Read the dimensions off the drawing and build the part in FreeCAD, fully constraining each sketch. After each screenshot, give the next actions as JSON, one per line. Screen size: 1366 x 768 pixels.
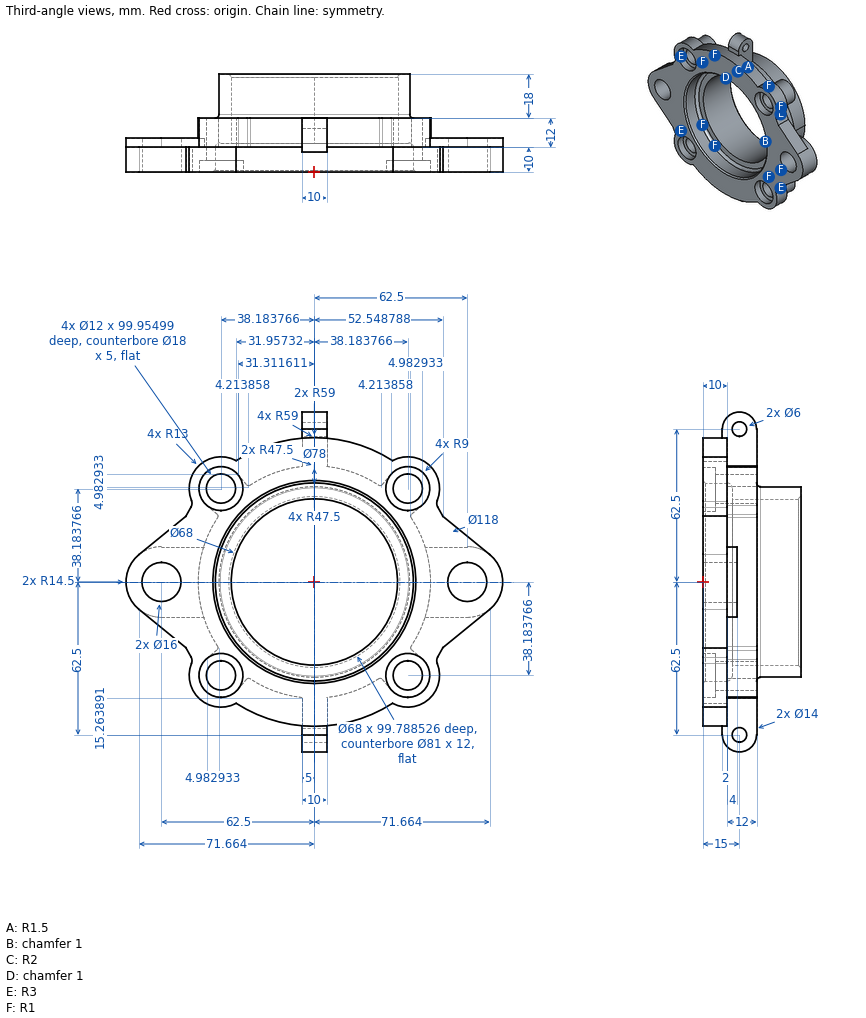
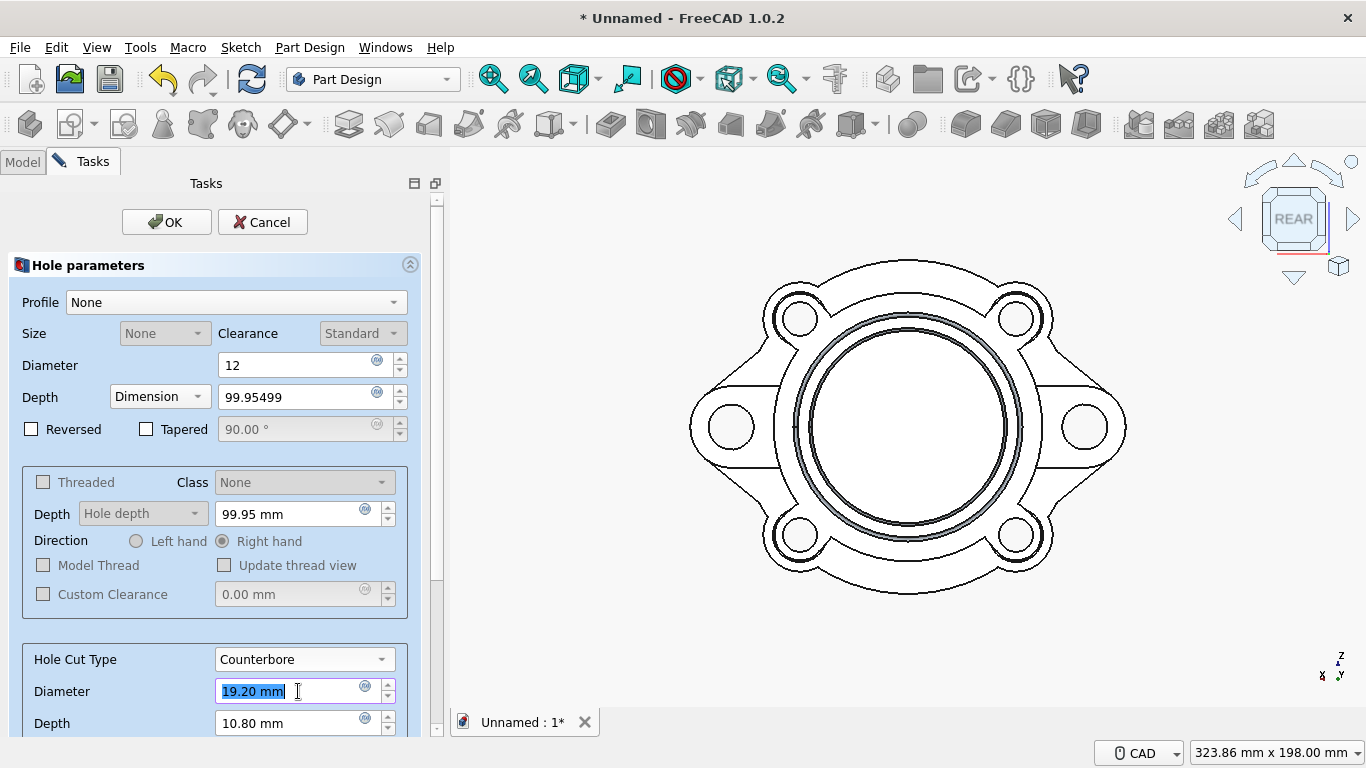
{"action": "type", "text": "18"}
{"action": "key", "text": "Tab"}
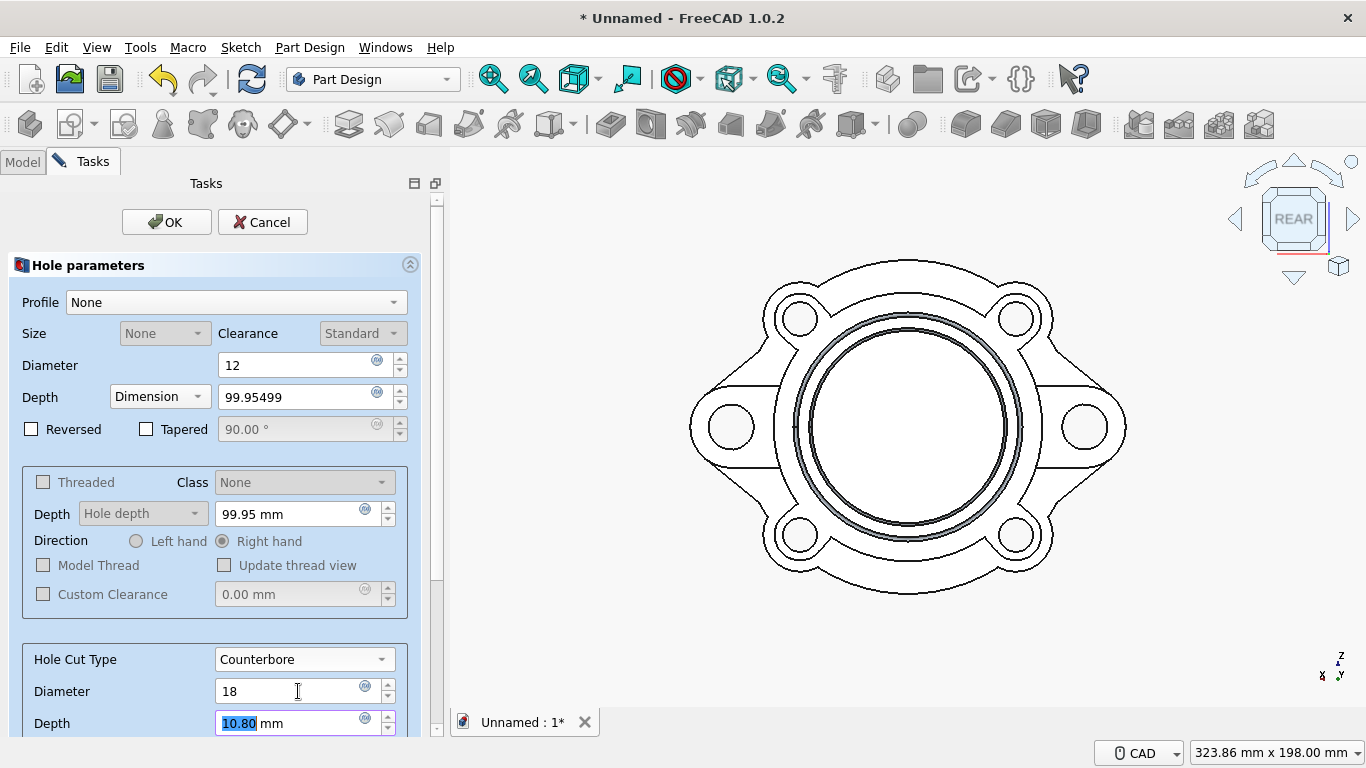
{"action": "type", "text": "5"}
{"action": "key", "text": "Tab"}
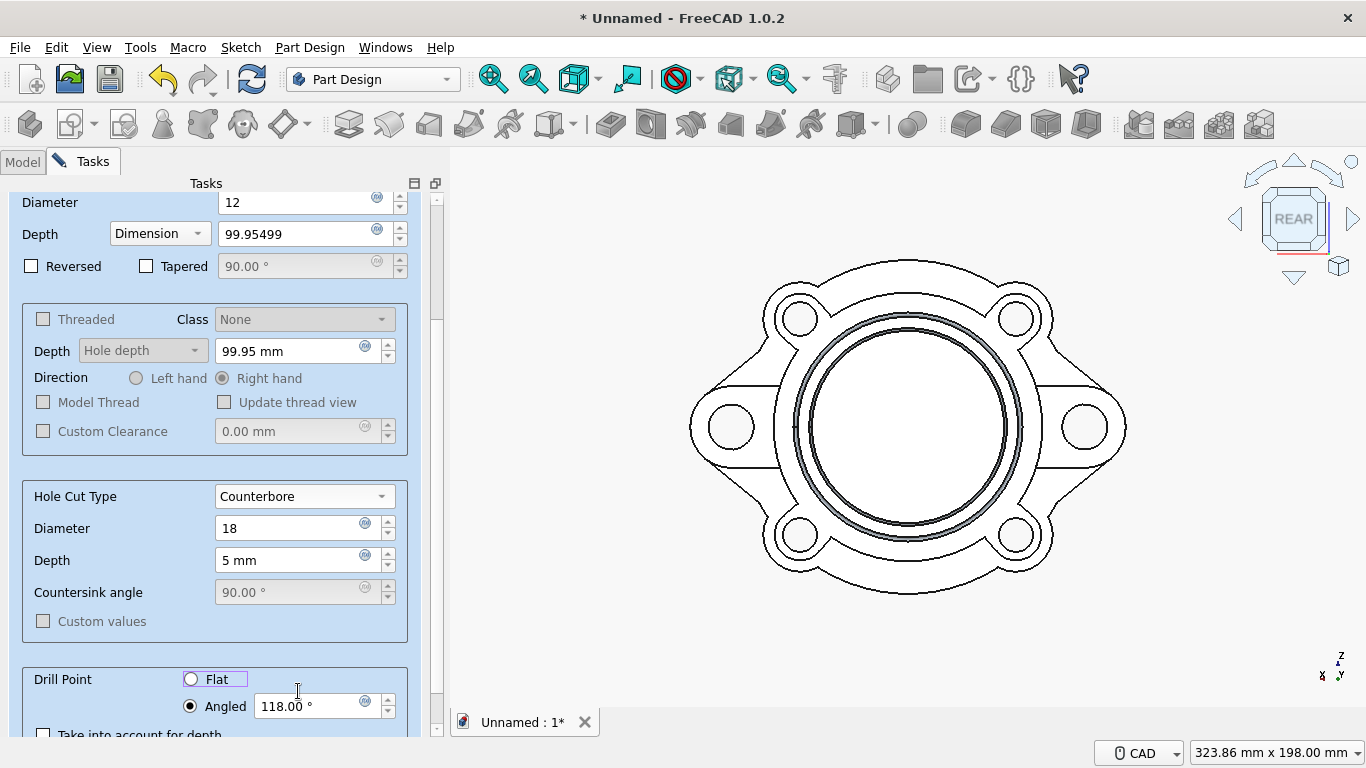
{"action": "left_click", "coordinate": [191, 679]}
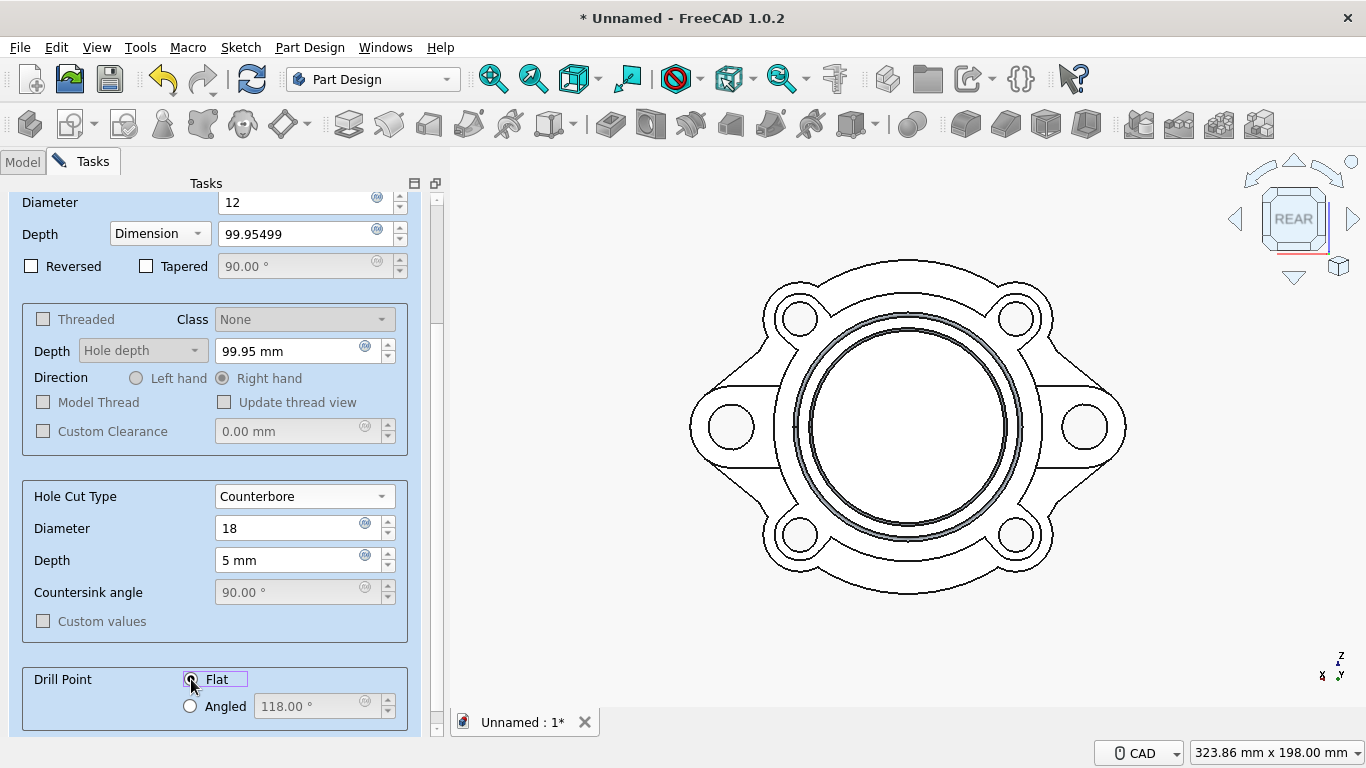
{"action": "scroll", "coordinate": [437, 464], "scroll_direction": "up", "scroll_amount": 4}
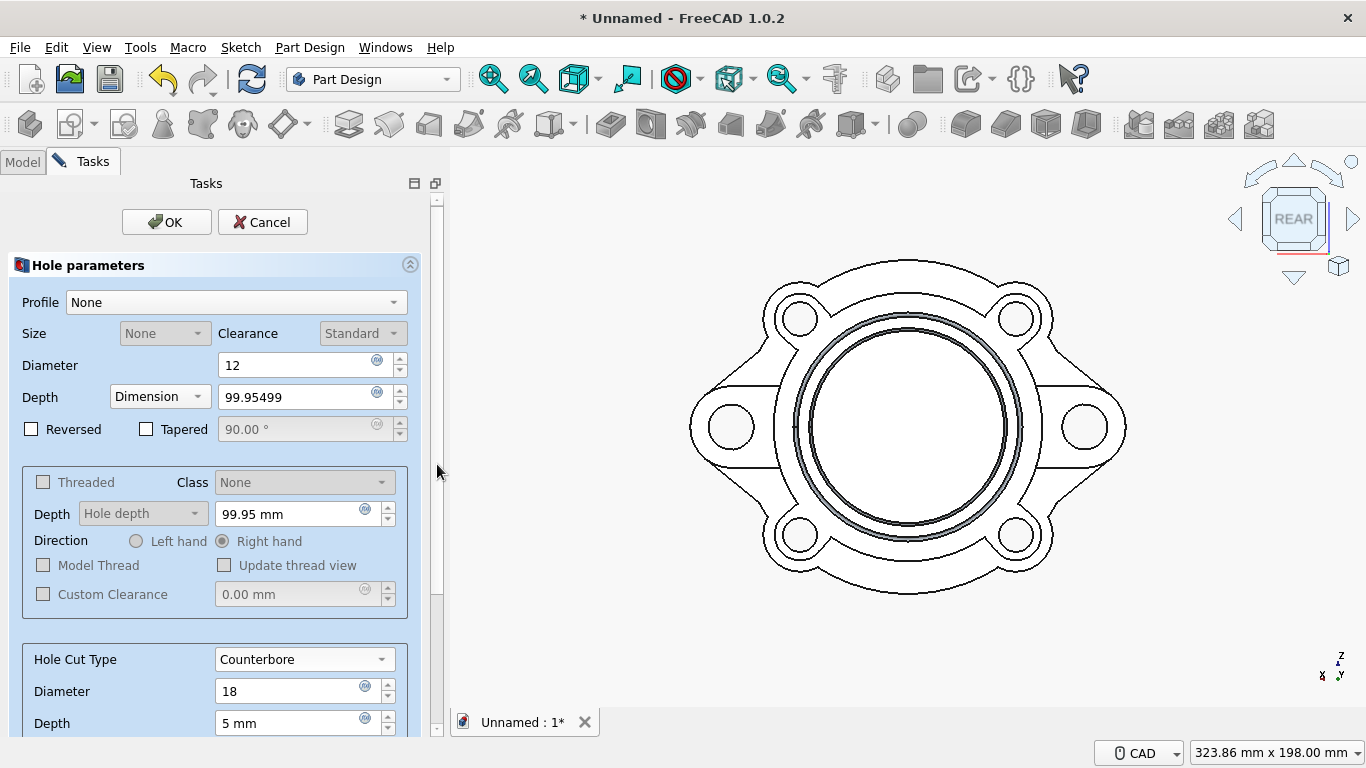
{"action": "left_click", "coordinate": [167, 222]}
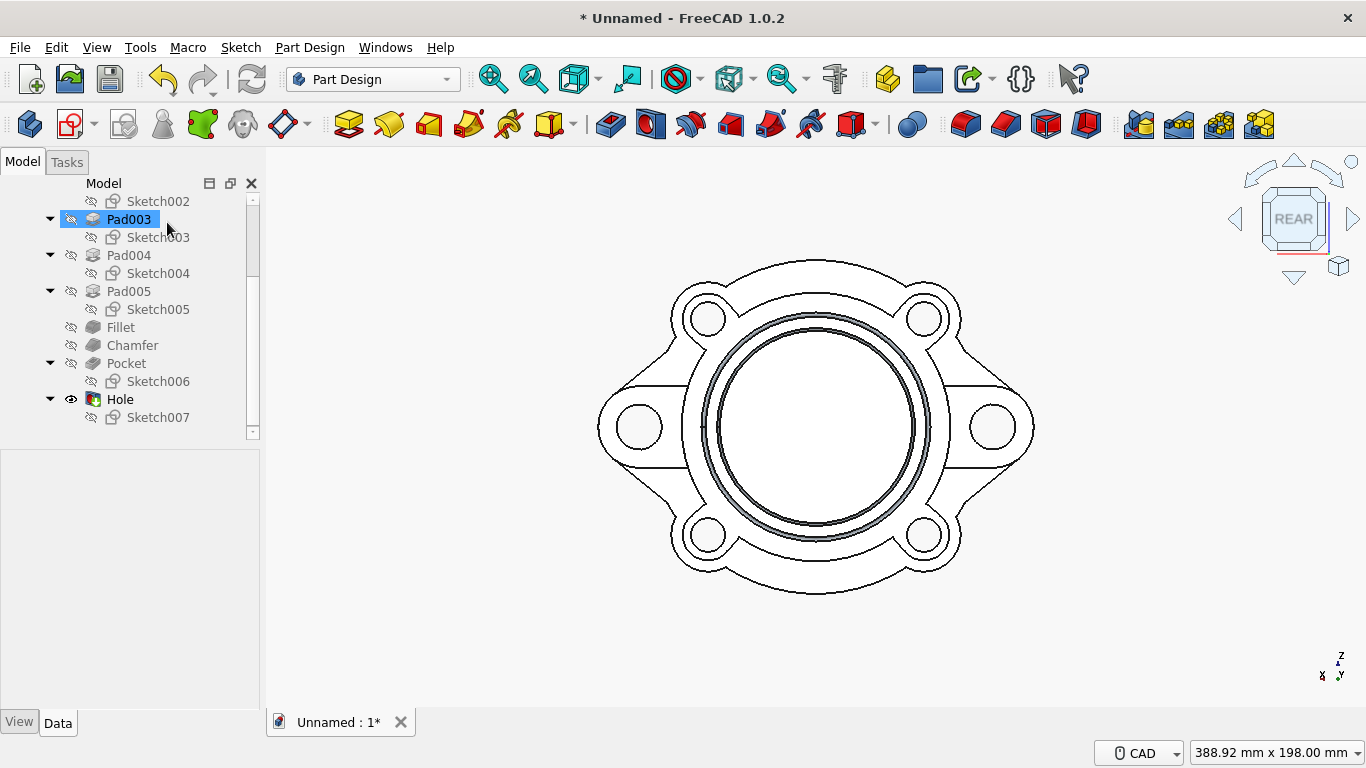
{"action": "left_click", "coordinate": [70, 124]}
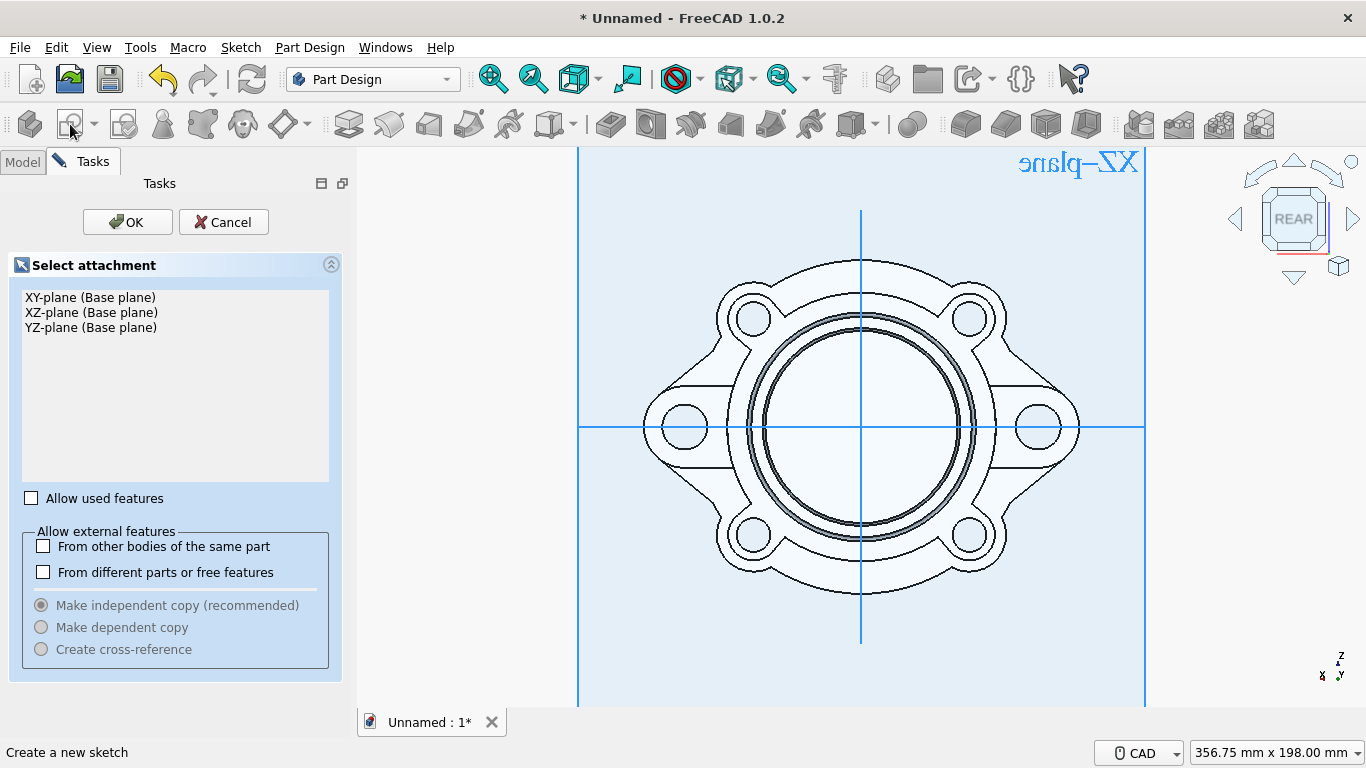
{"action": "left_click", "coordinate": [82, 312]}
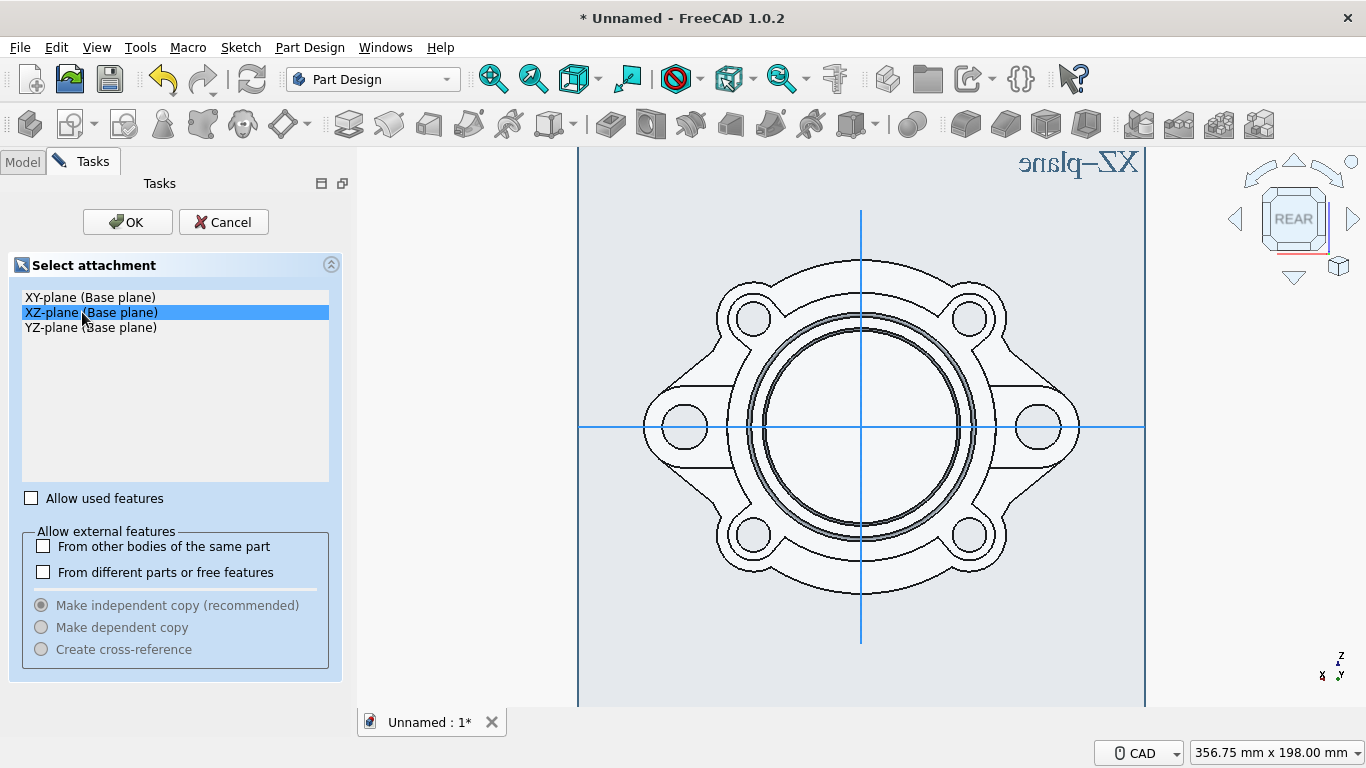
{"action": "left_click", "coordinate": [128, 222]}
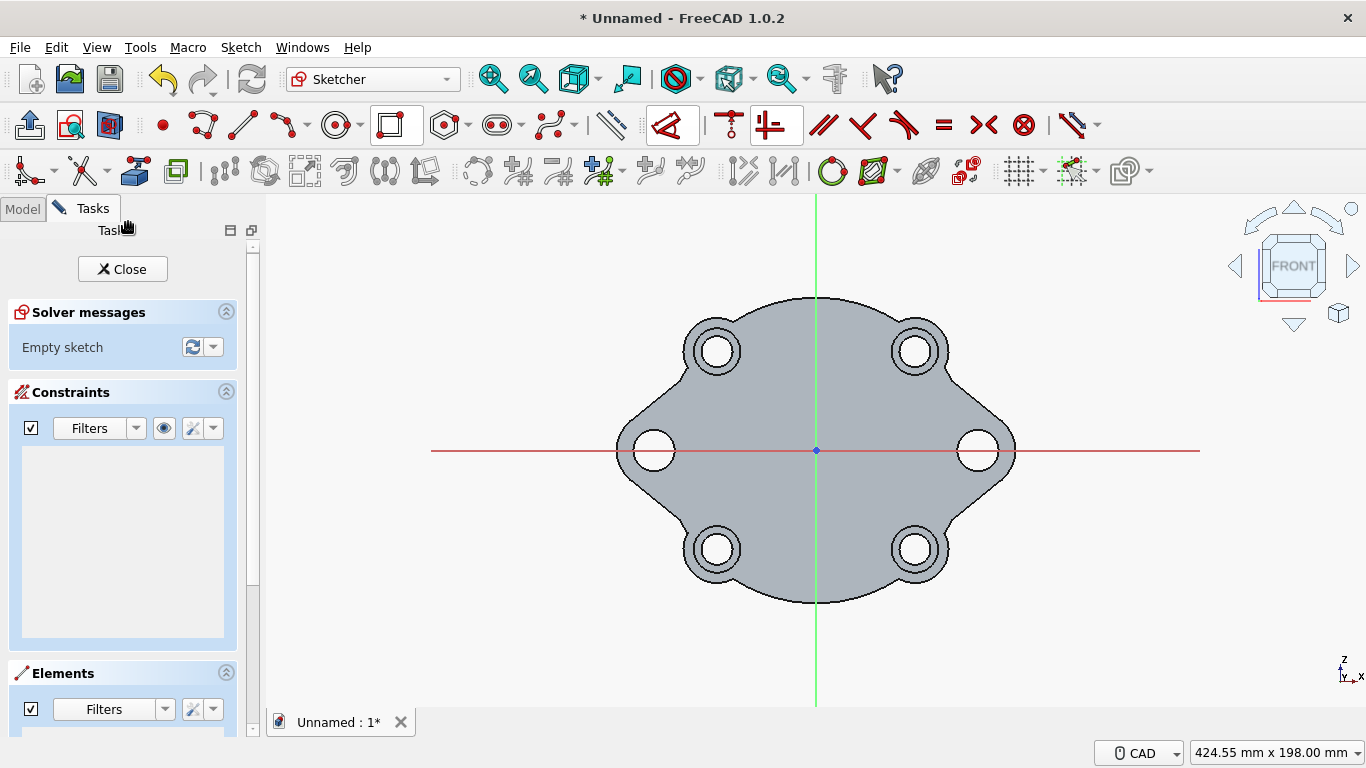
{"action": "scroll", "coordinate": [899, 451], "scroll_direction": "up", "scroll_amount": 3}